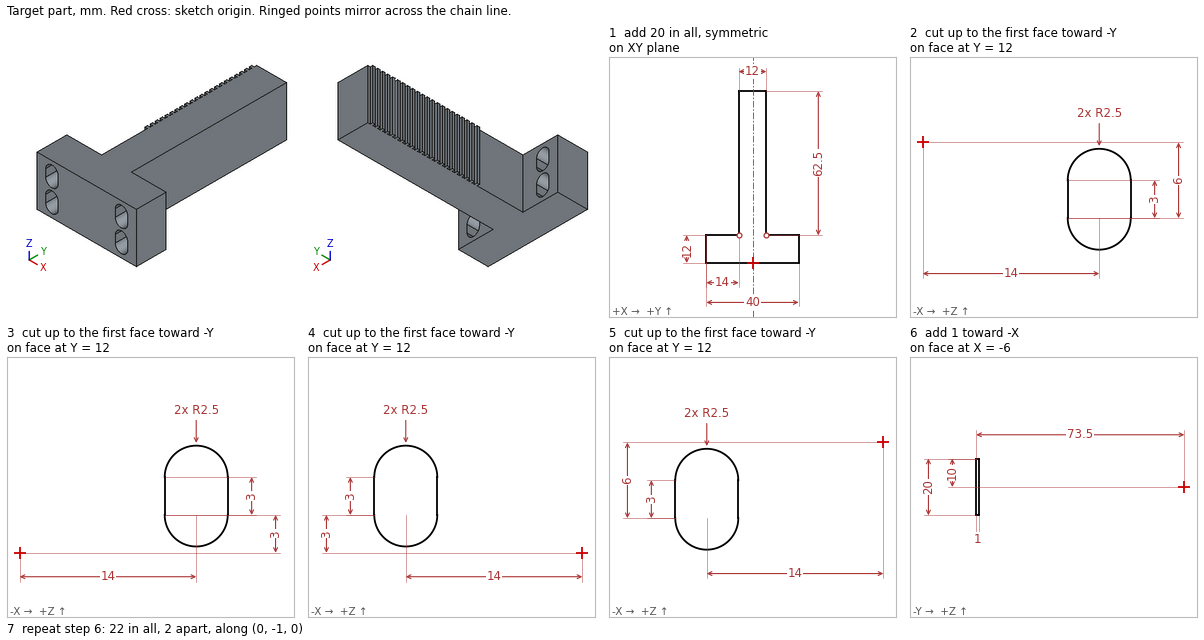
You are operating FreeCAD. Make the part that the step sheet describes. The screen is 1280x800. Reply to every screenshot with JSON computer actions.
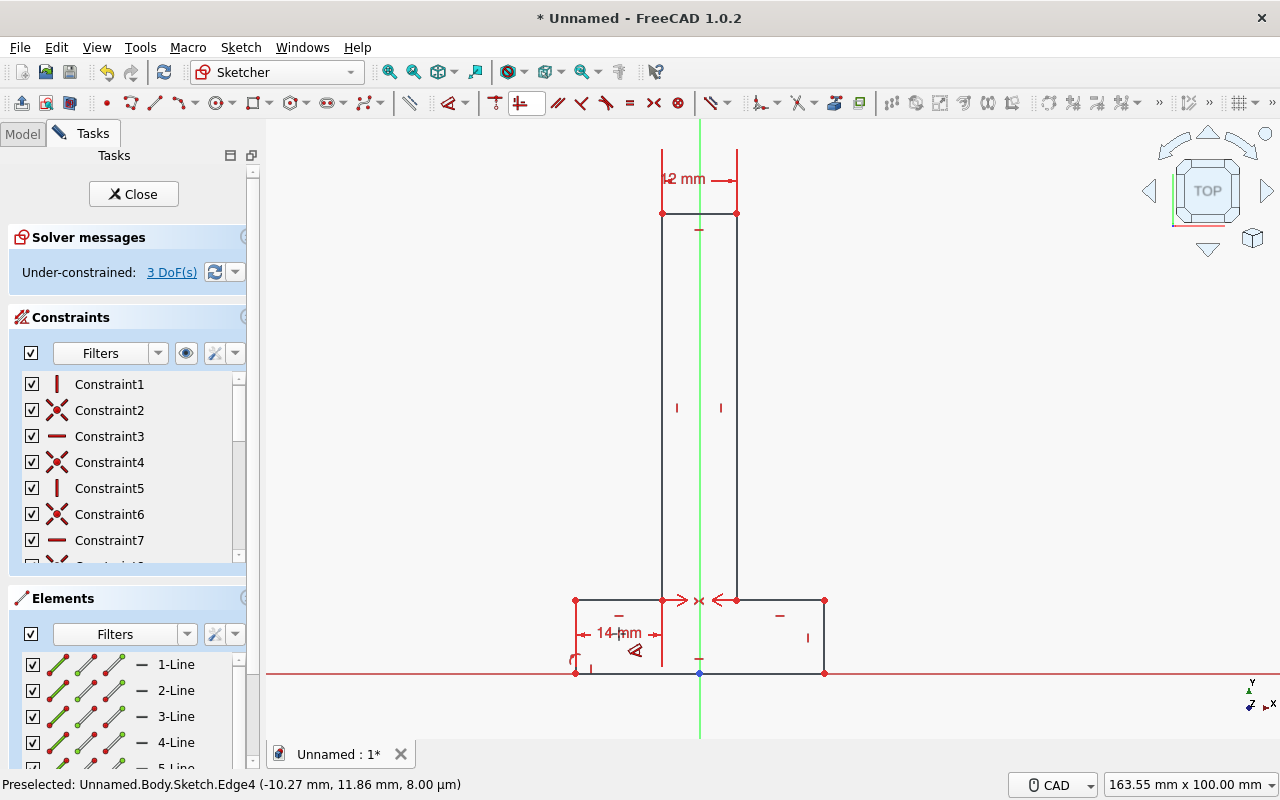
{"action": "left_click", "coordinate": [576, 622]}
{"action": "left_click", "coordinate": [542, 637]}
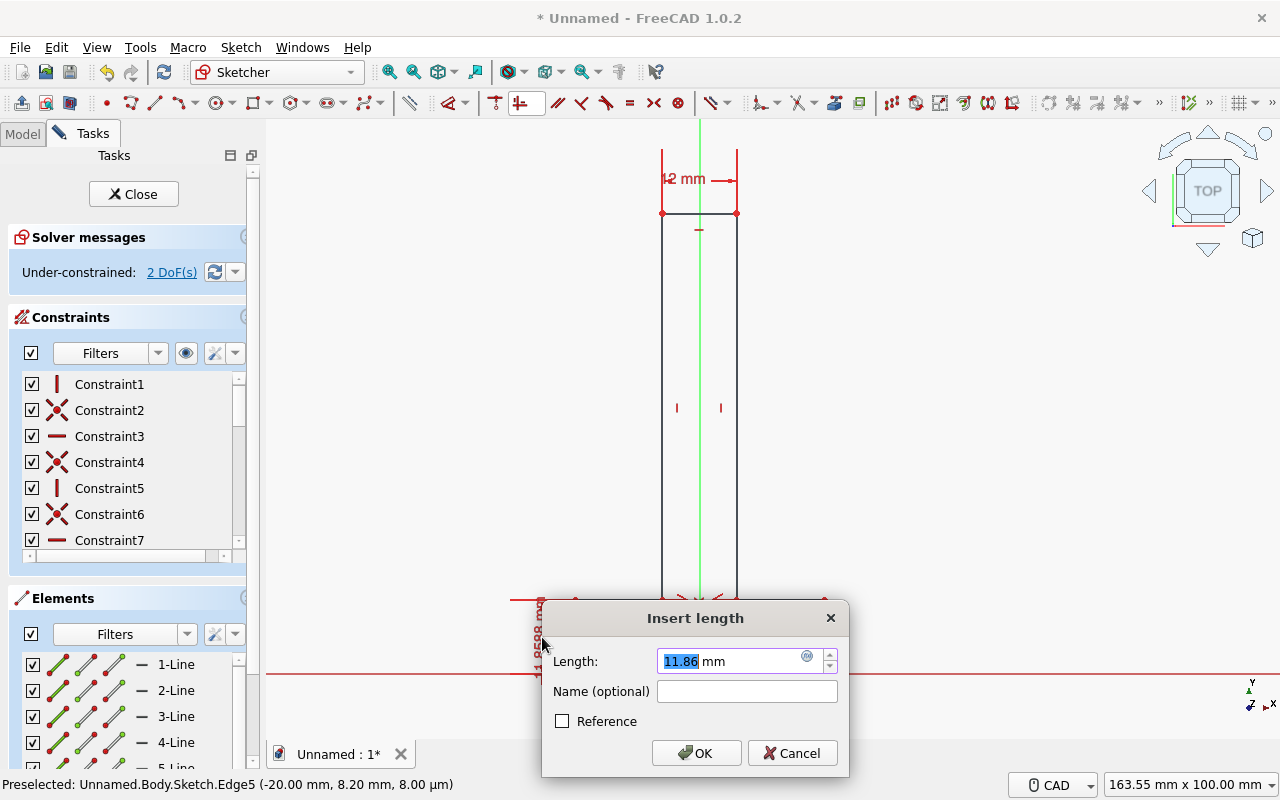
{"action": "type", "text": "12"}
{"action": "key", "text": "Return"}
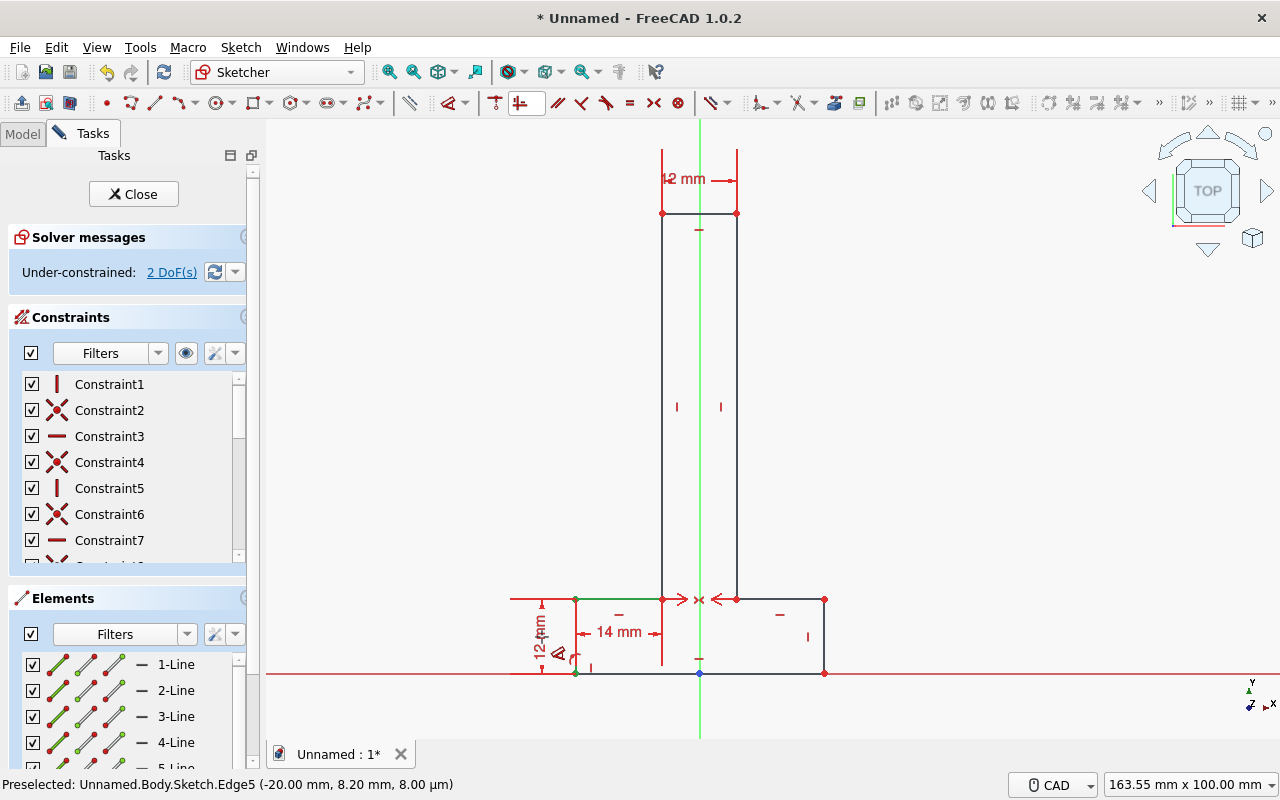
{"action": "left_click", "coordinate": [650, 674]}
{"action": "left_click", "coordinate": [643, 708]}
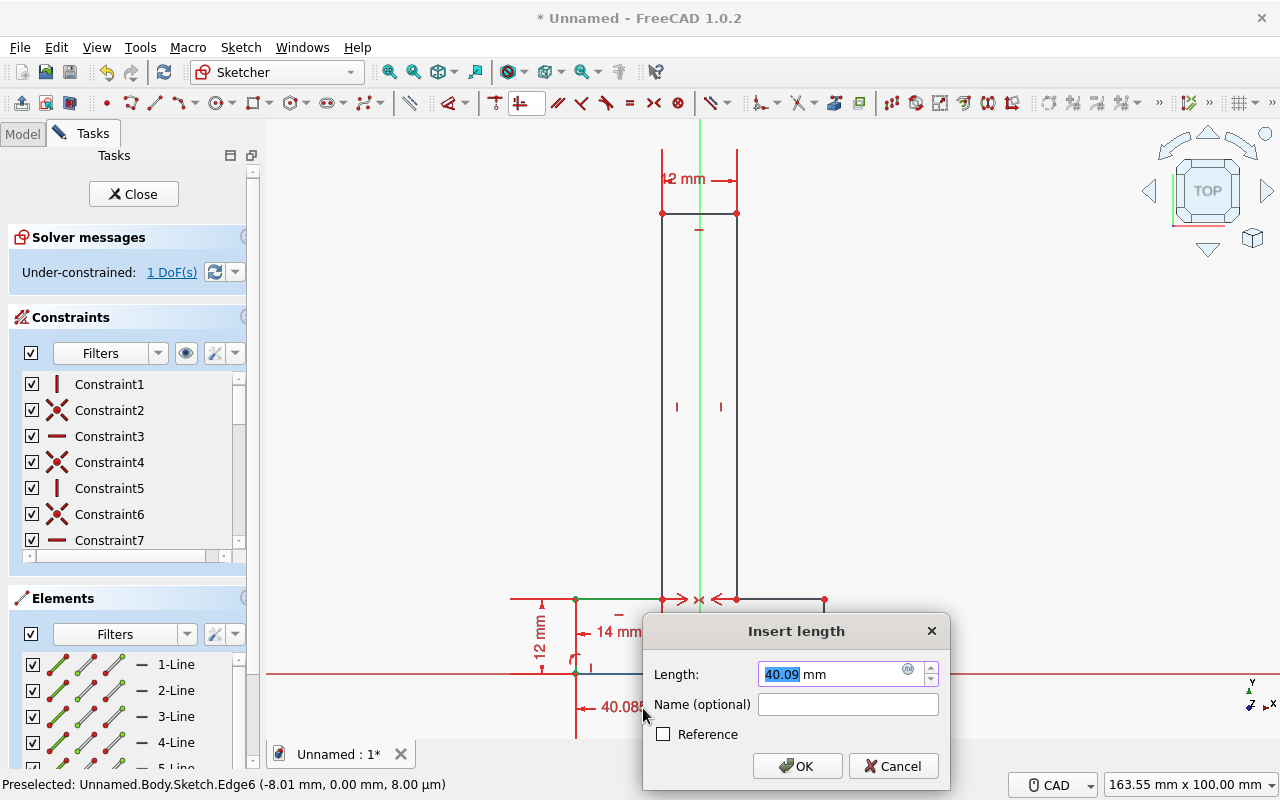
{"action": "type", "text": "40"}
{"action": "key", "text": "Return"}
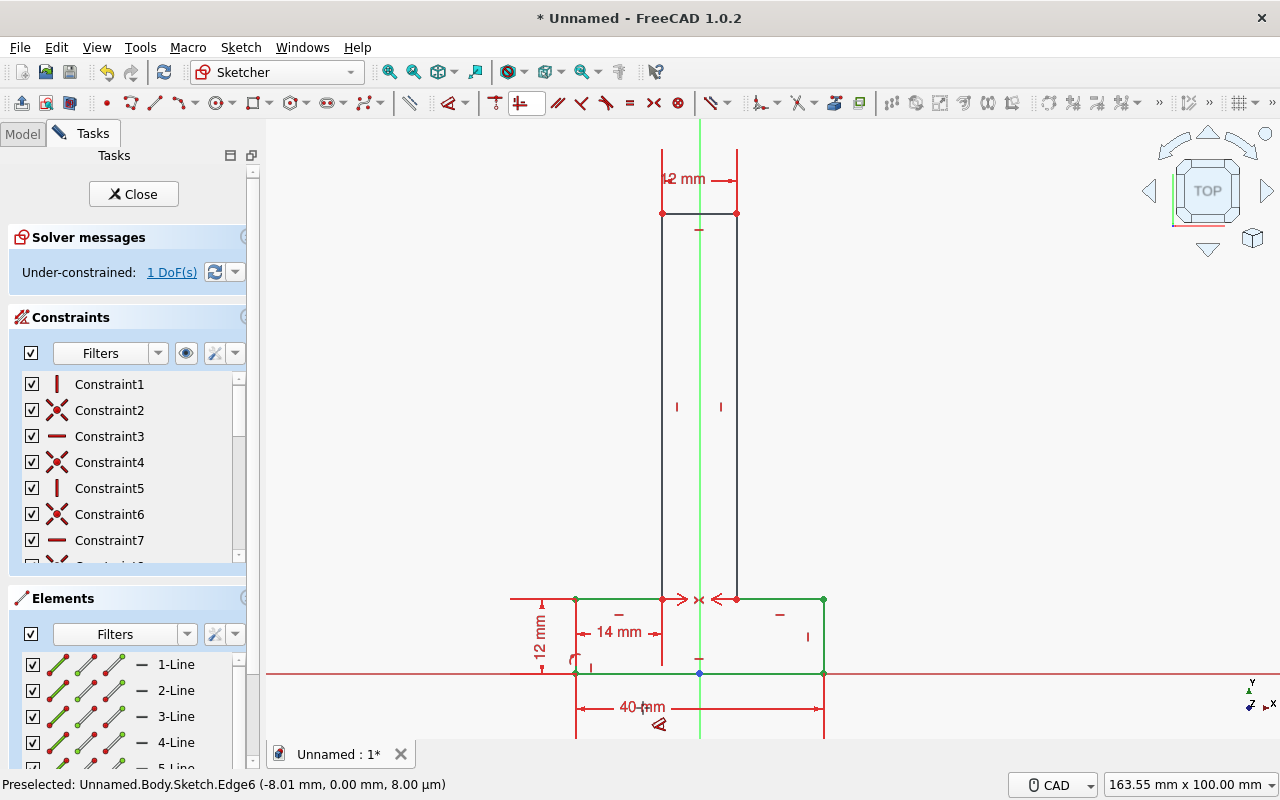
{"action": "left_click", "coordinate": [737, 484]}
{"action": "left_click", "coordinate": [771, 407]}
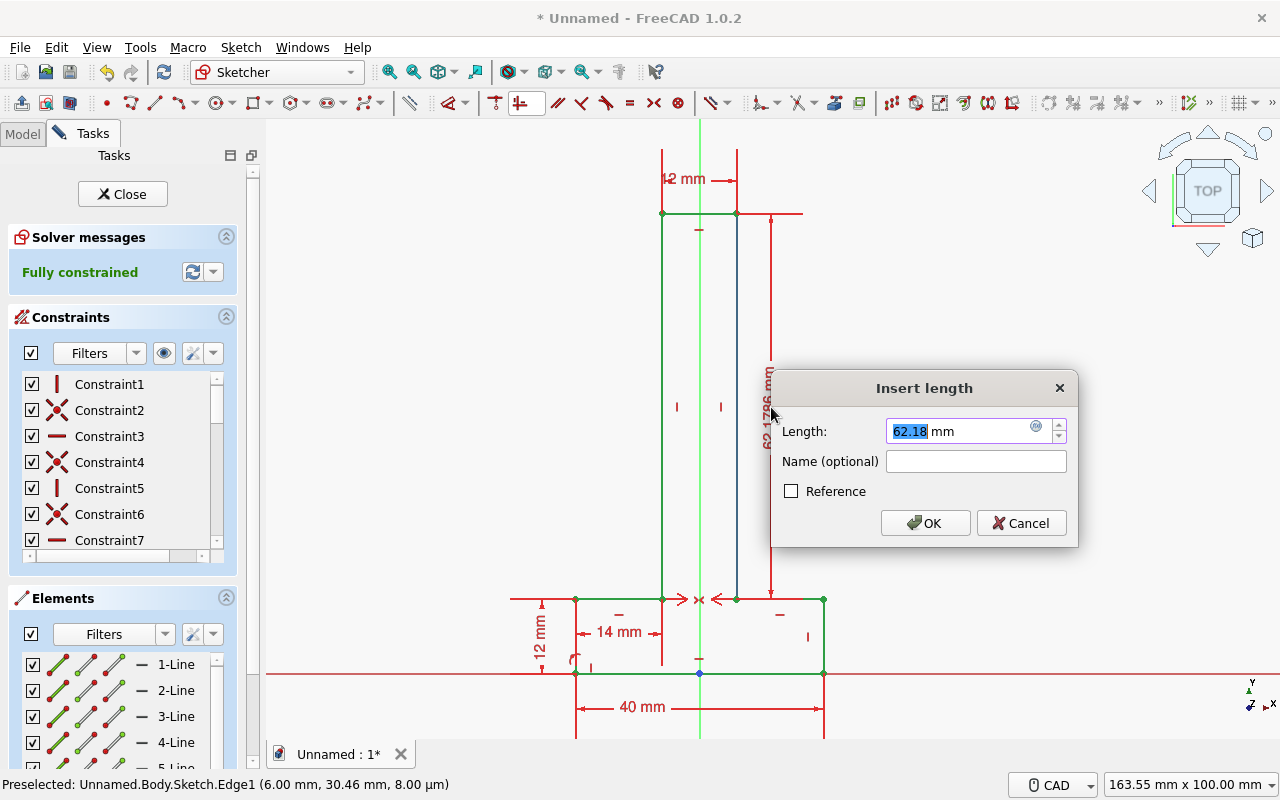
{"action": "type", "text": "62.5"}
{"action": "key", "text": "Return"}
{"action": "key", "text": "Escape"}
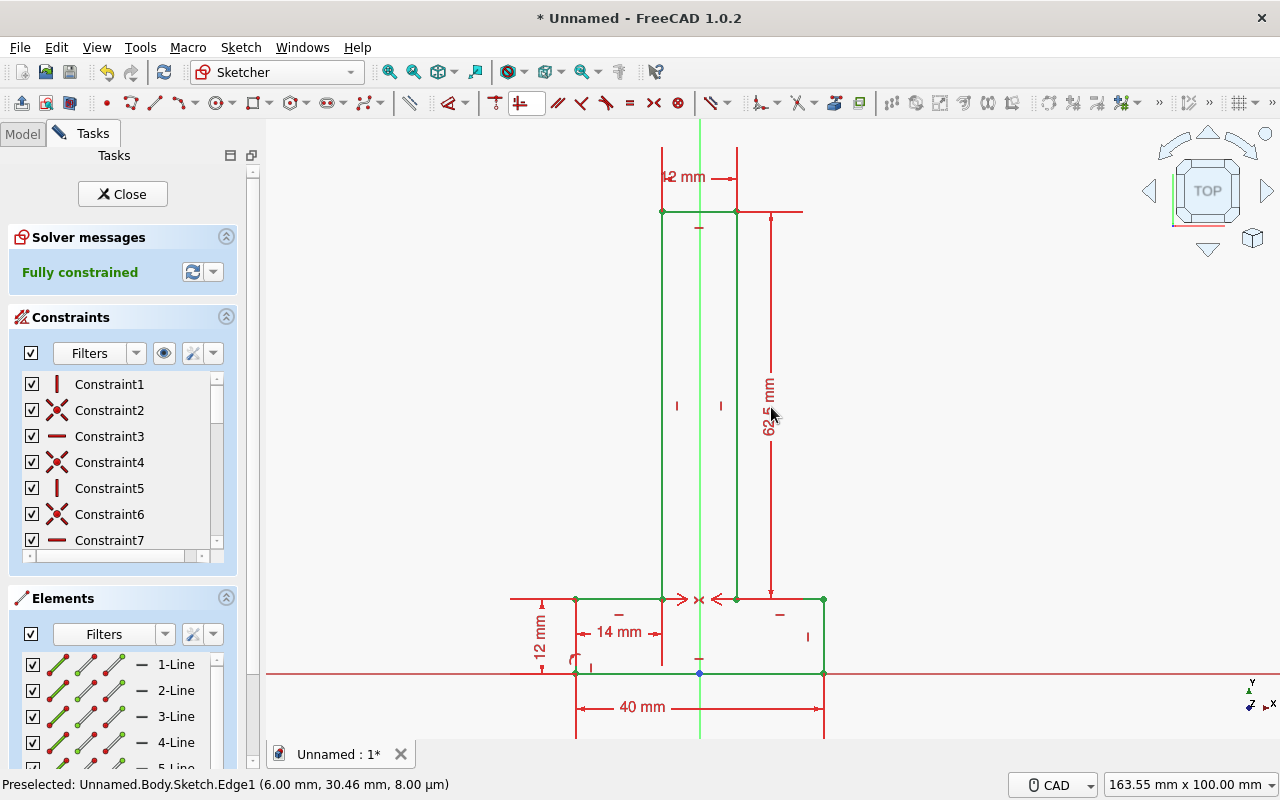
{"action": "left_click", "coordinate": [123, 194]}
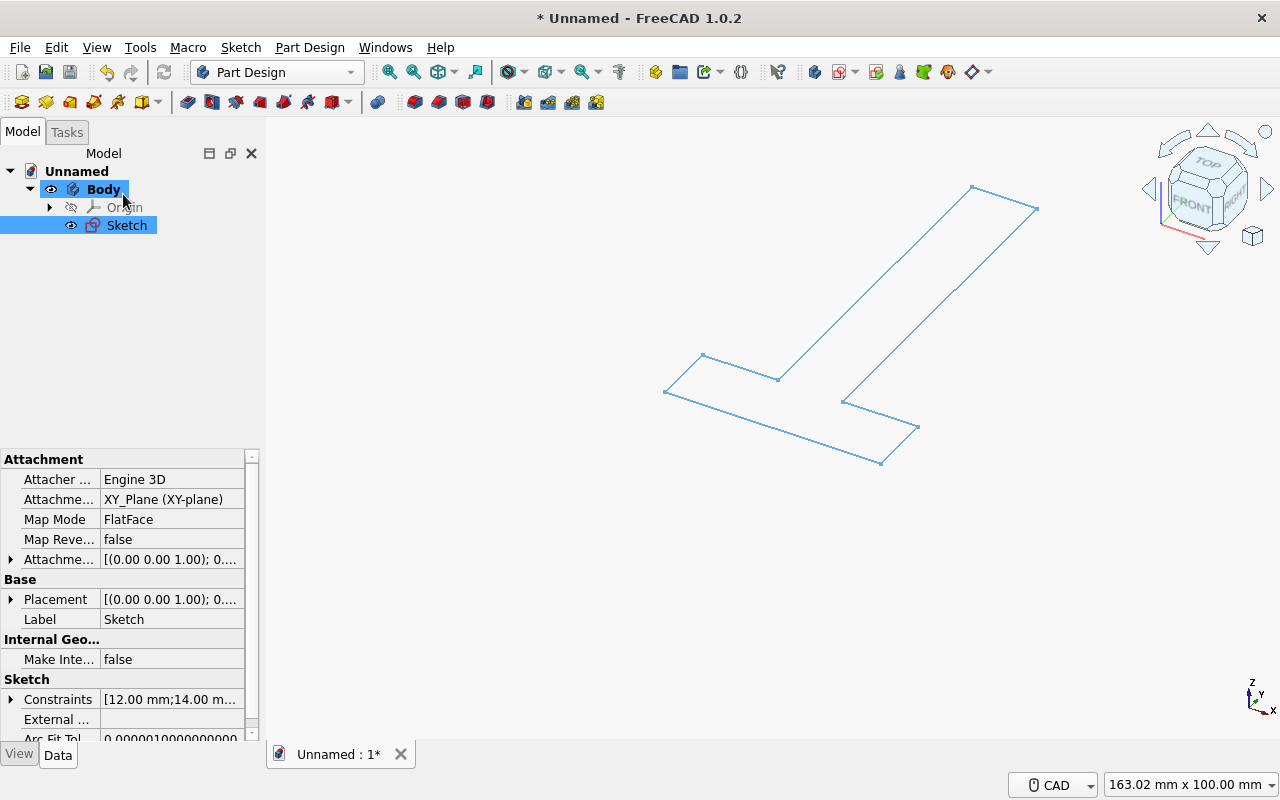
{"action": "left_click", "coordinate": [22, 102]}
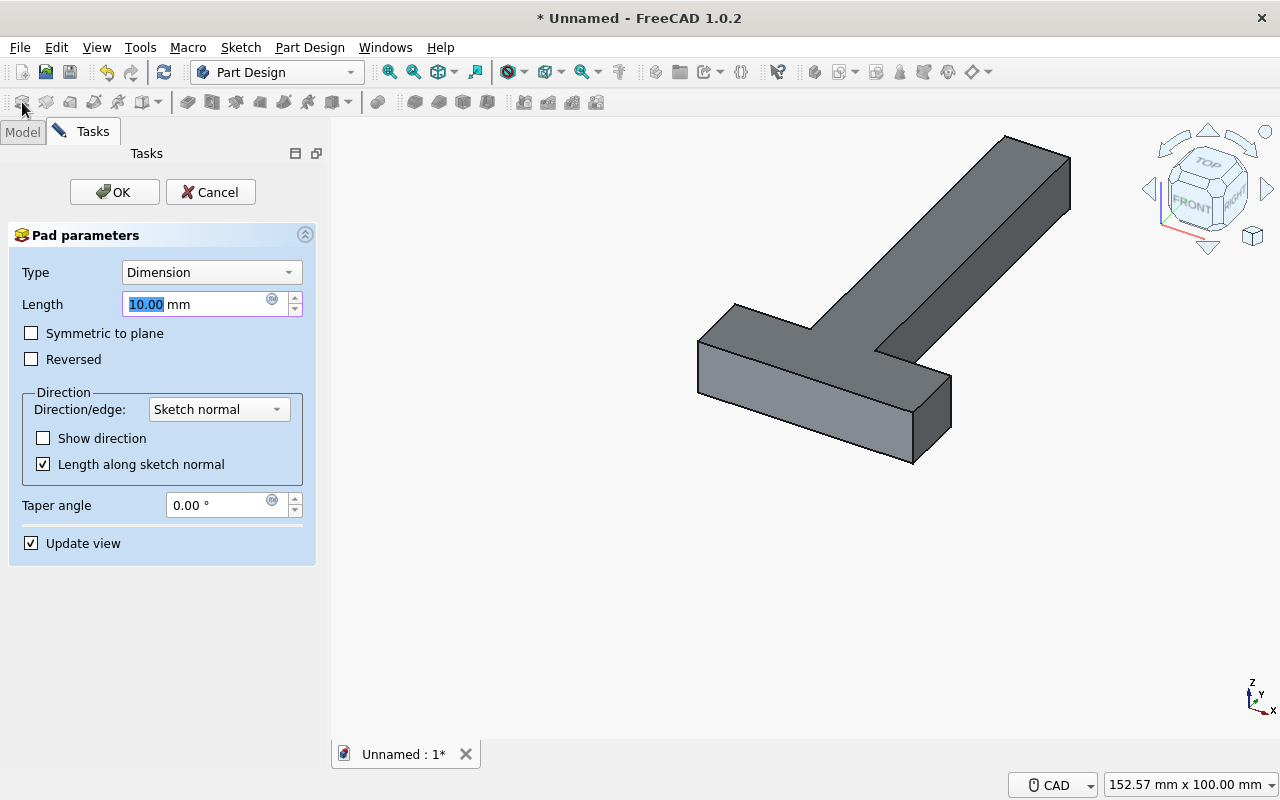
{"action": "type", "text": "20"}
{"action": "key", "text": "Tab"}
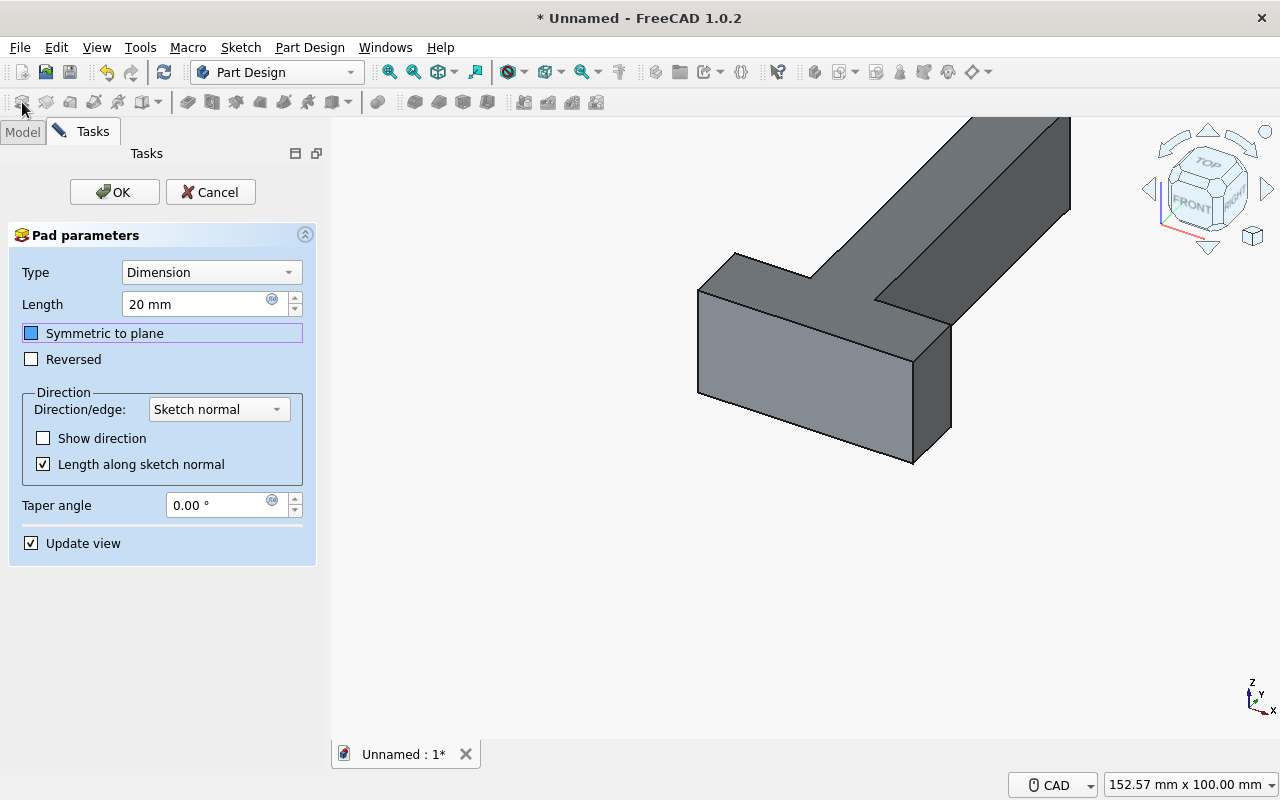
{"action": "left_click", "coordinate": [30, 333]}